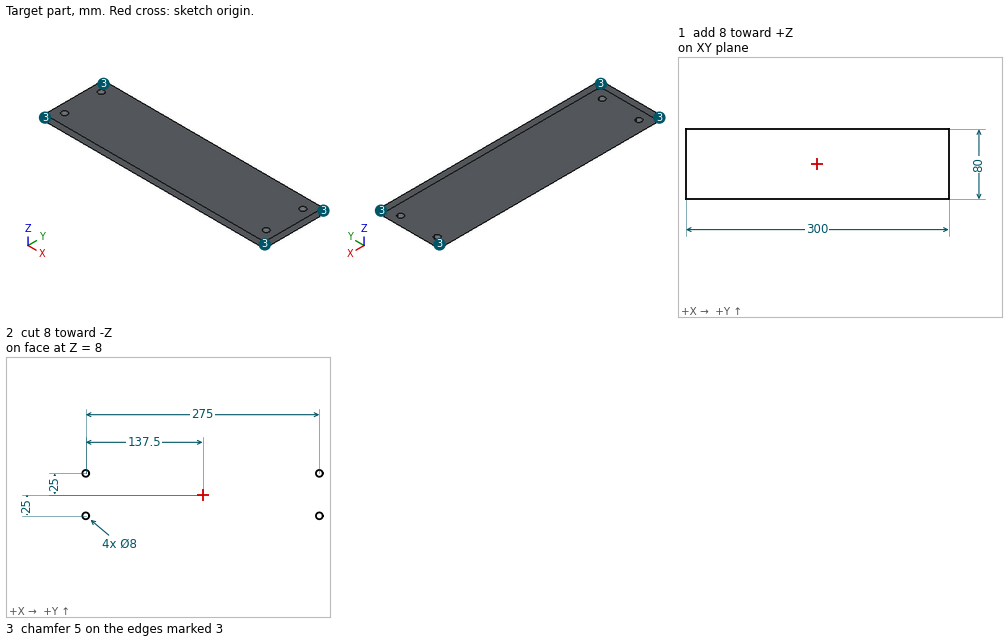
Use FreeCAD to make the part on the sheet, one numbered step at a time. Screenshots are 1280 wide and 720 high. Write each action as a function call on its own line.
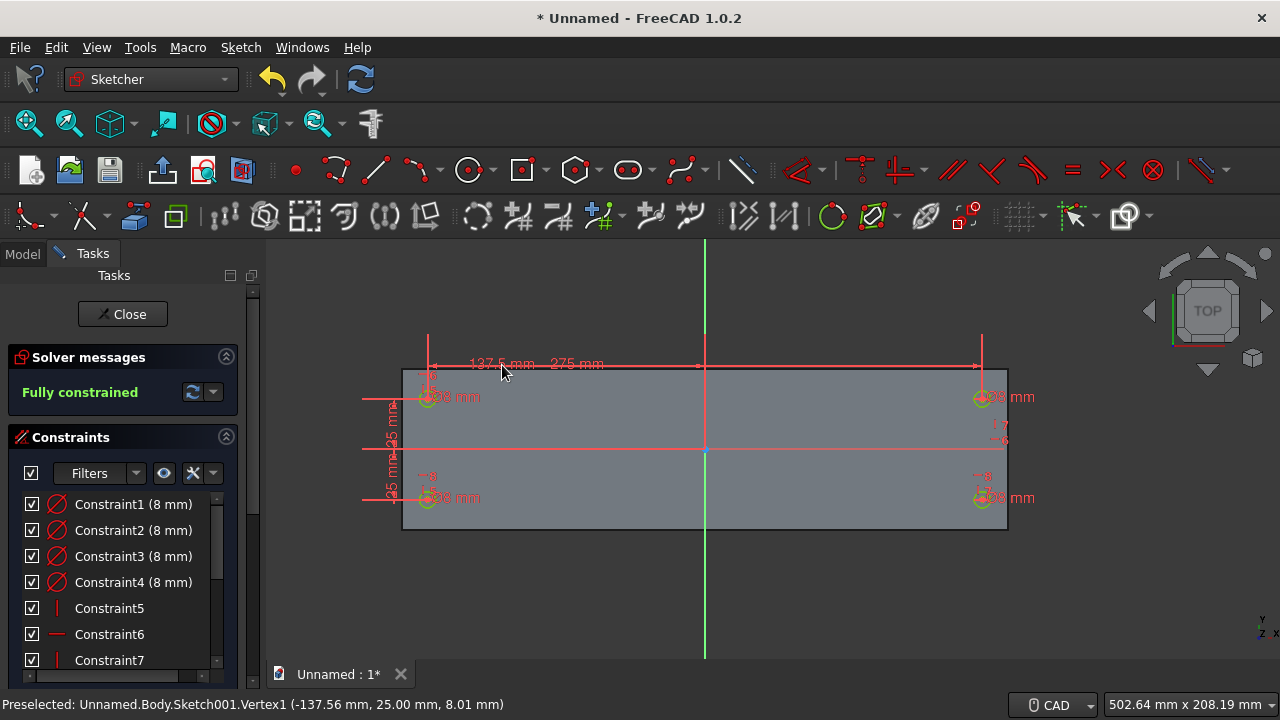
click(123, 314)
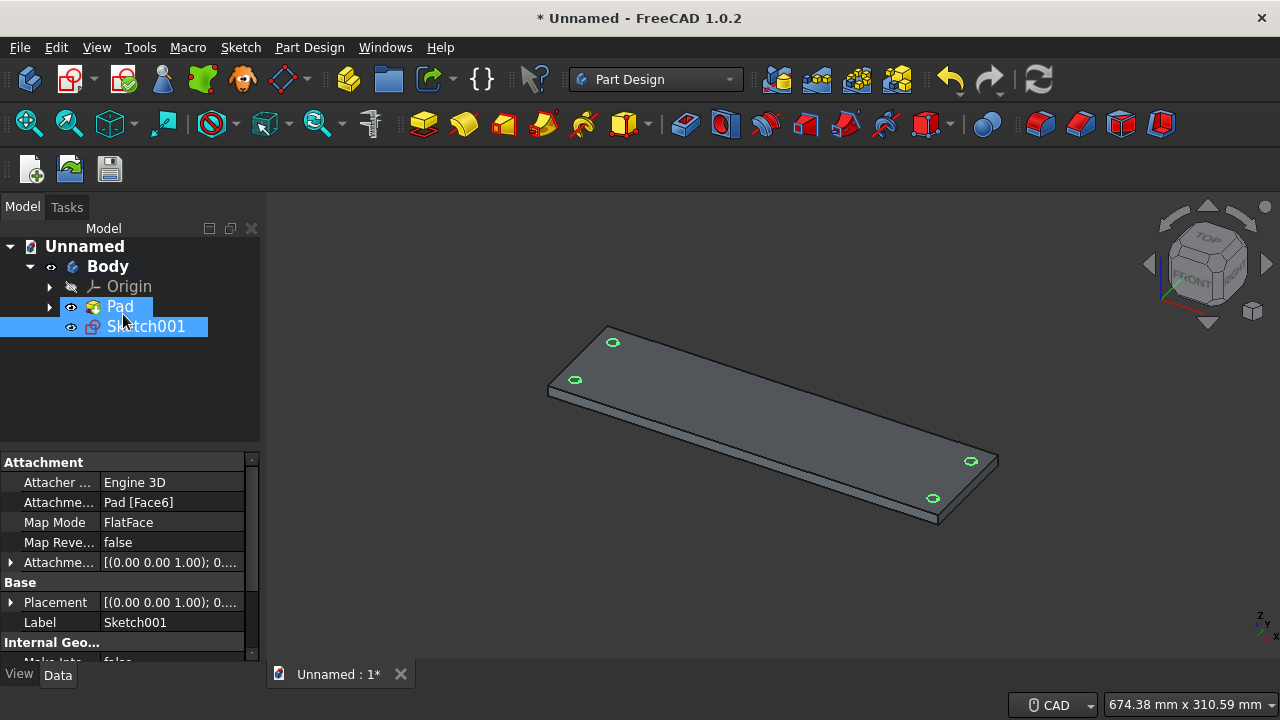
click(686, 124)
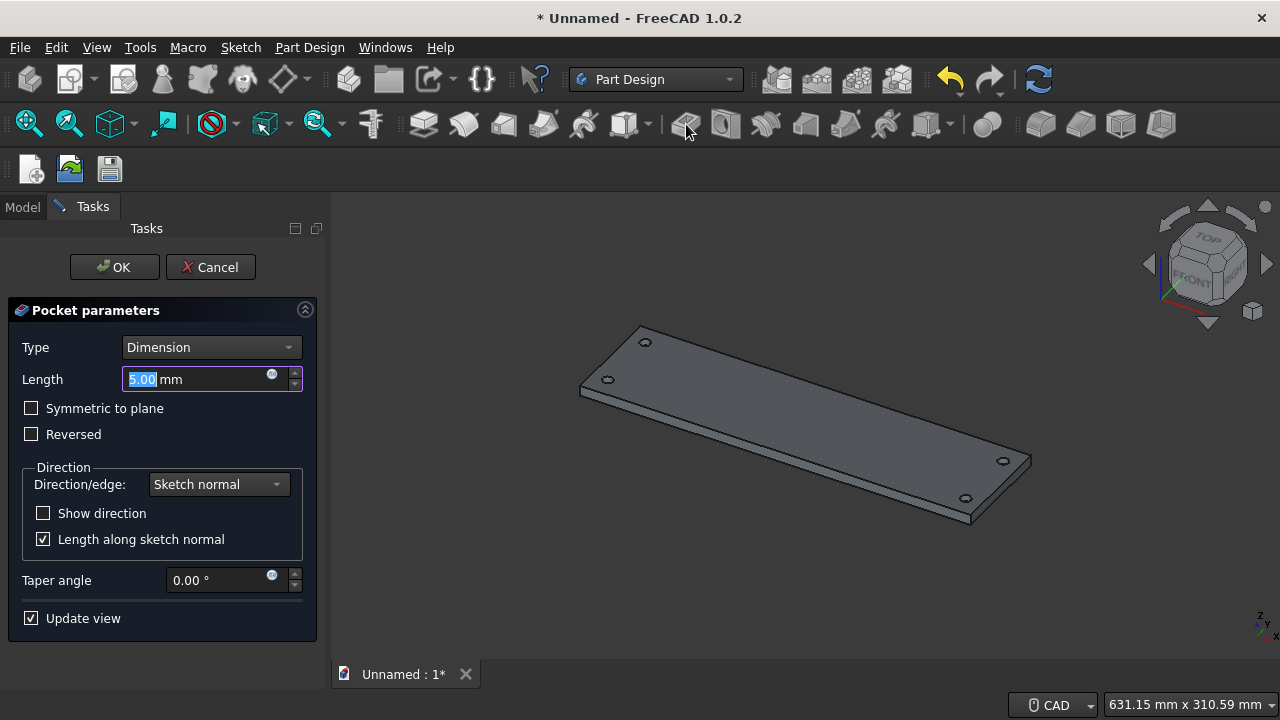
text(8)
key(Tab)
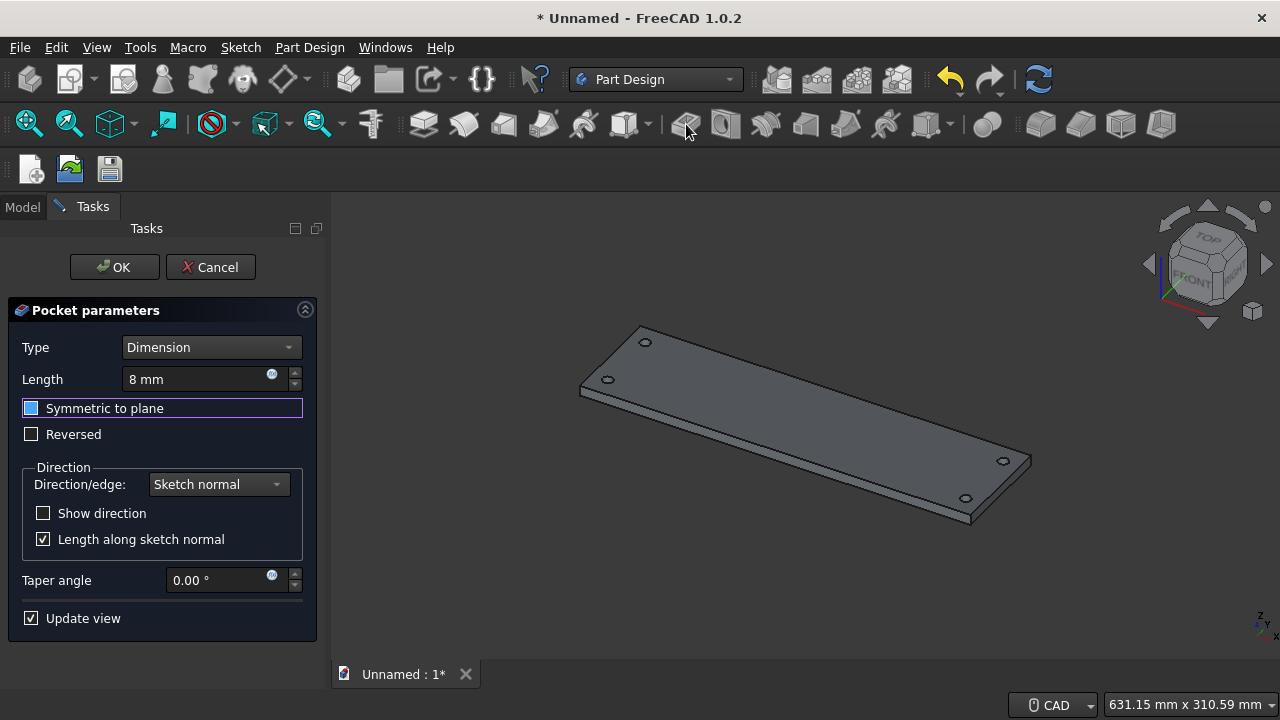
click(115, 267)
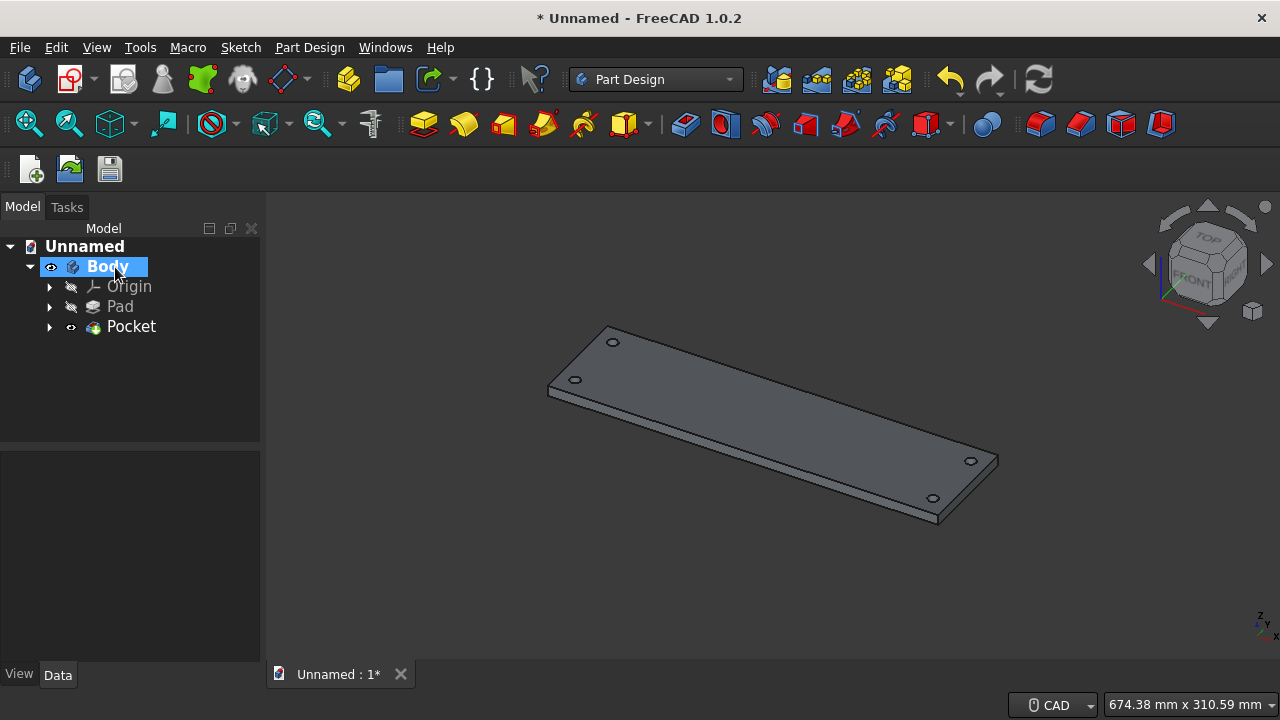
key(v)
key(f)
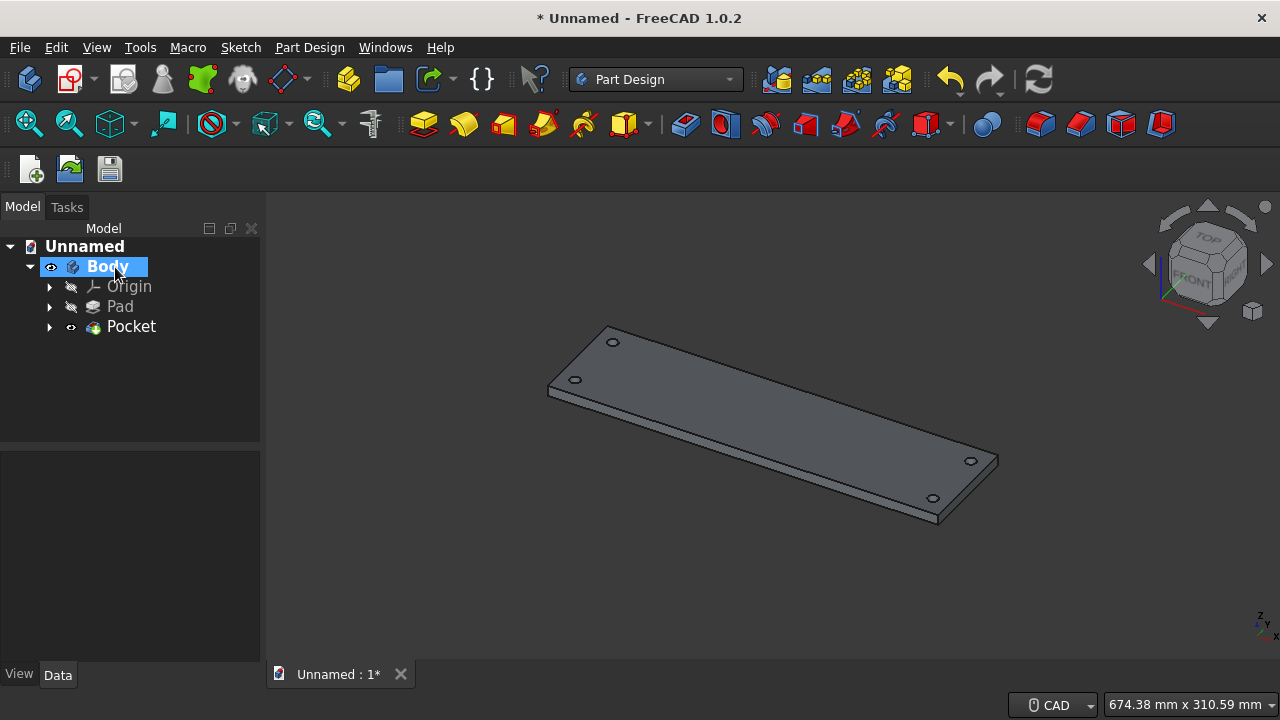
click(938, 521)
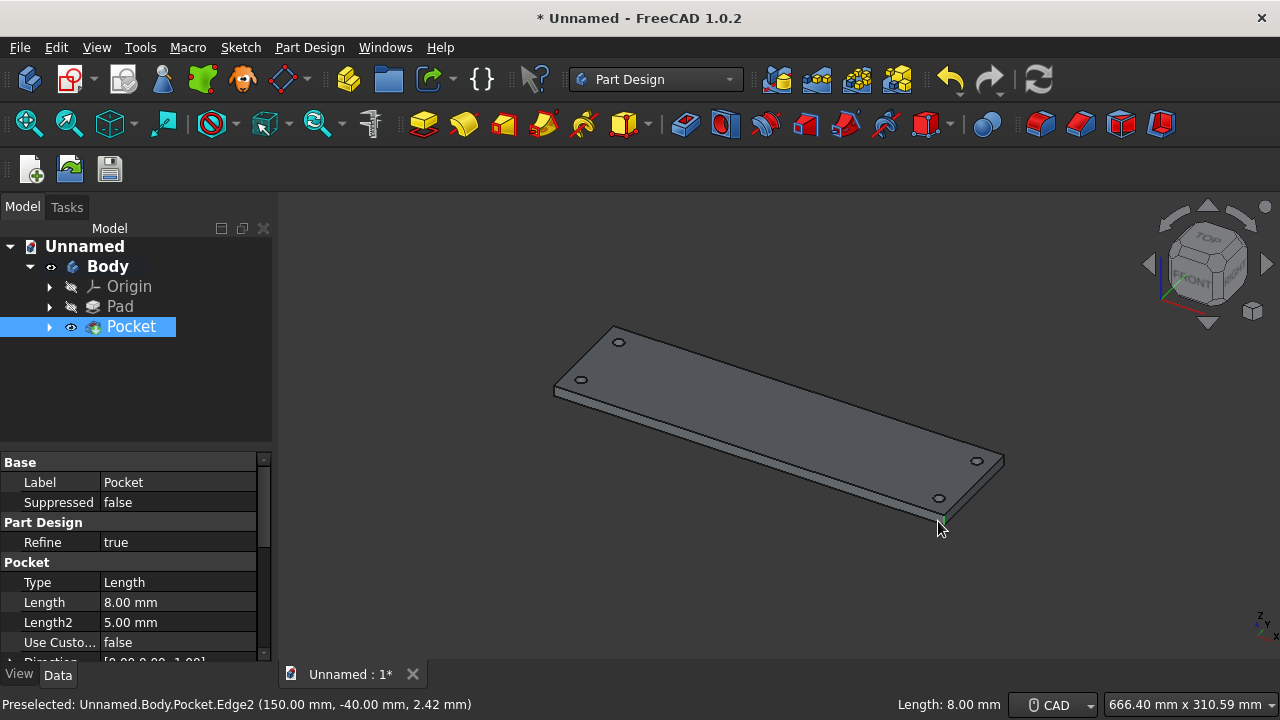
scroll(554, 390, up, 7)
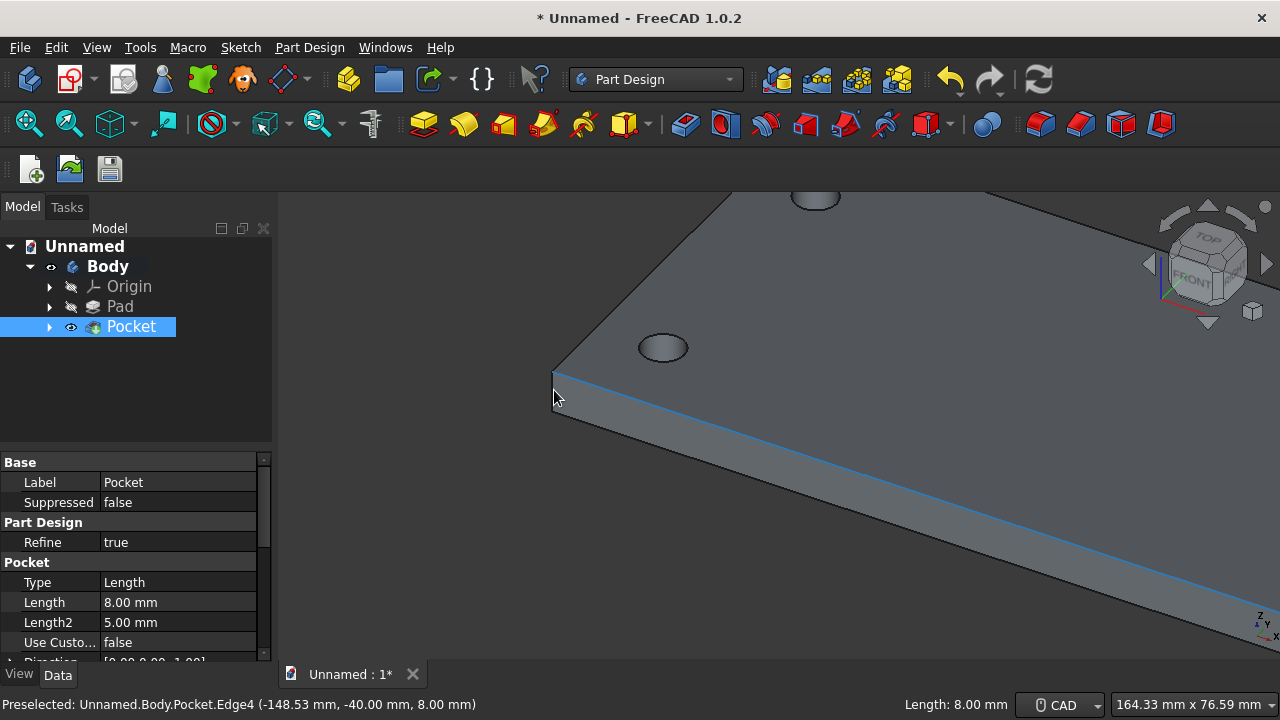
key(v)
key(f)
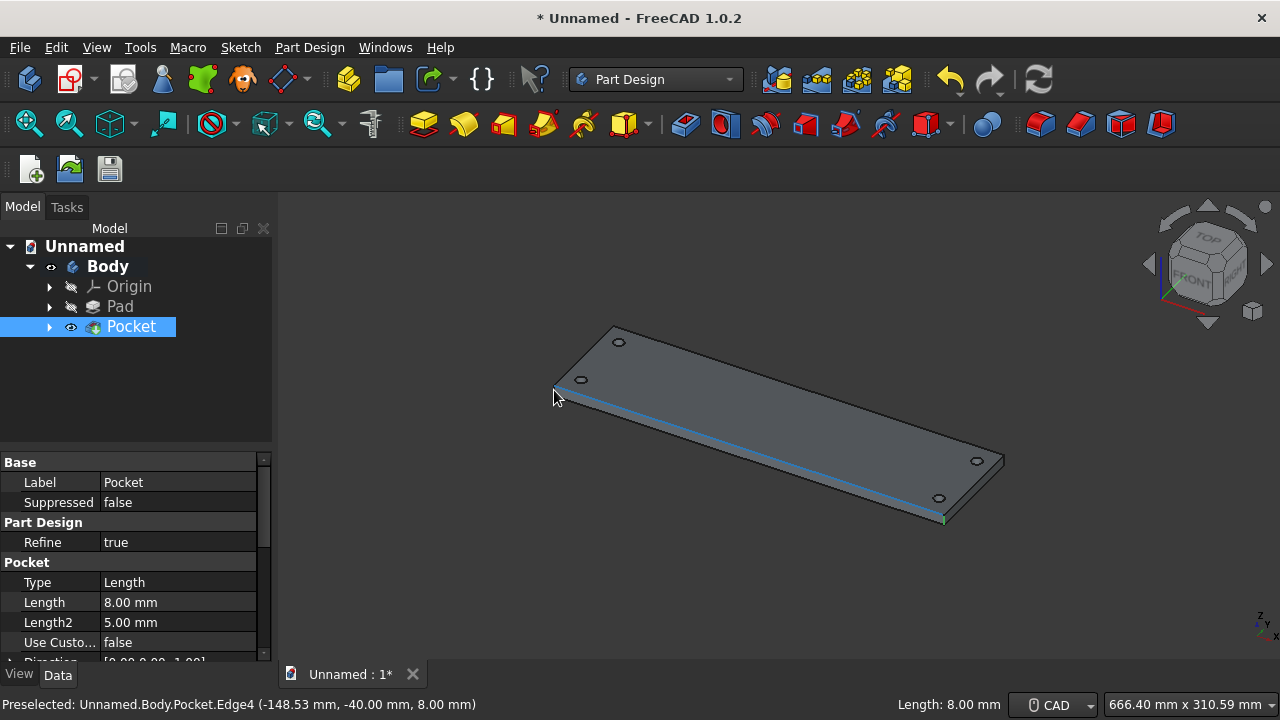
key(0)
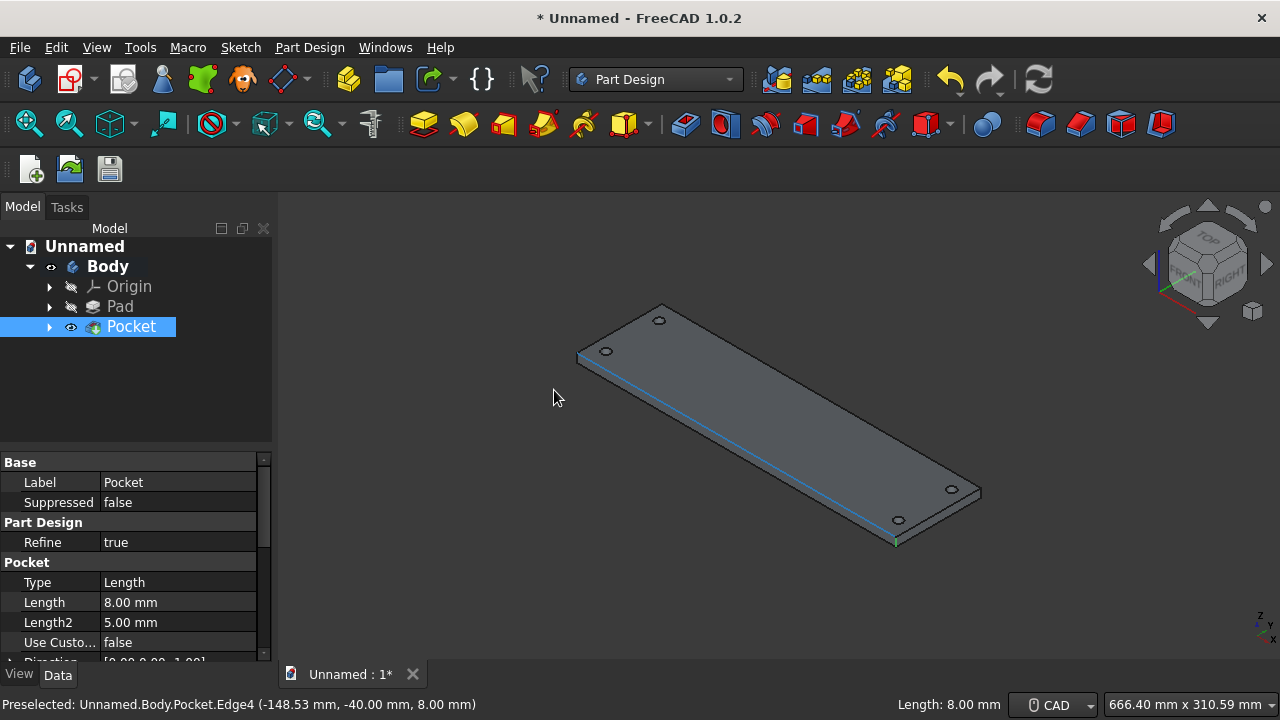
scroll(577, 357, up, 7)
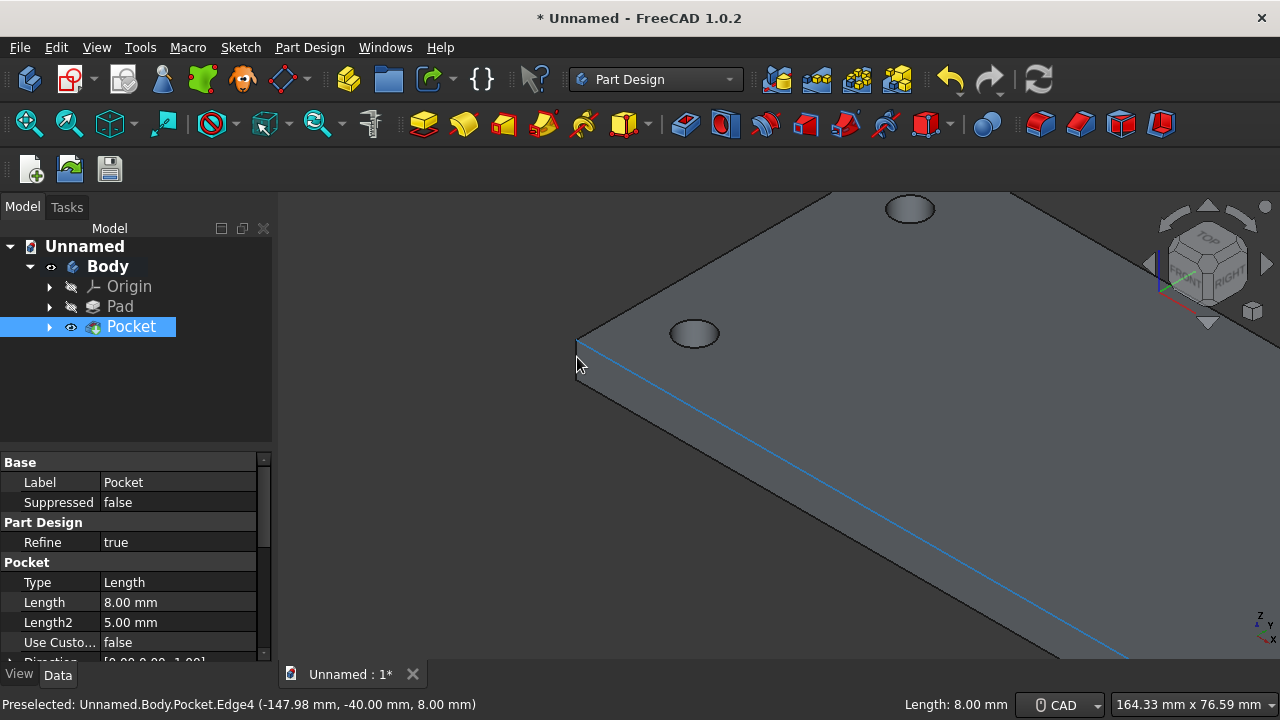
key(v)
key(f)